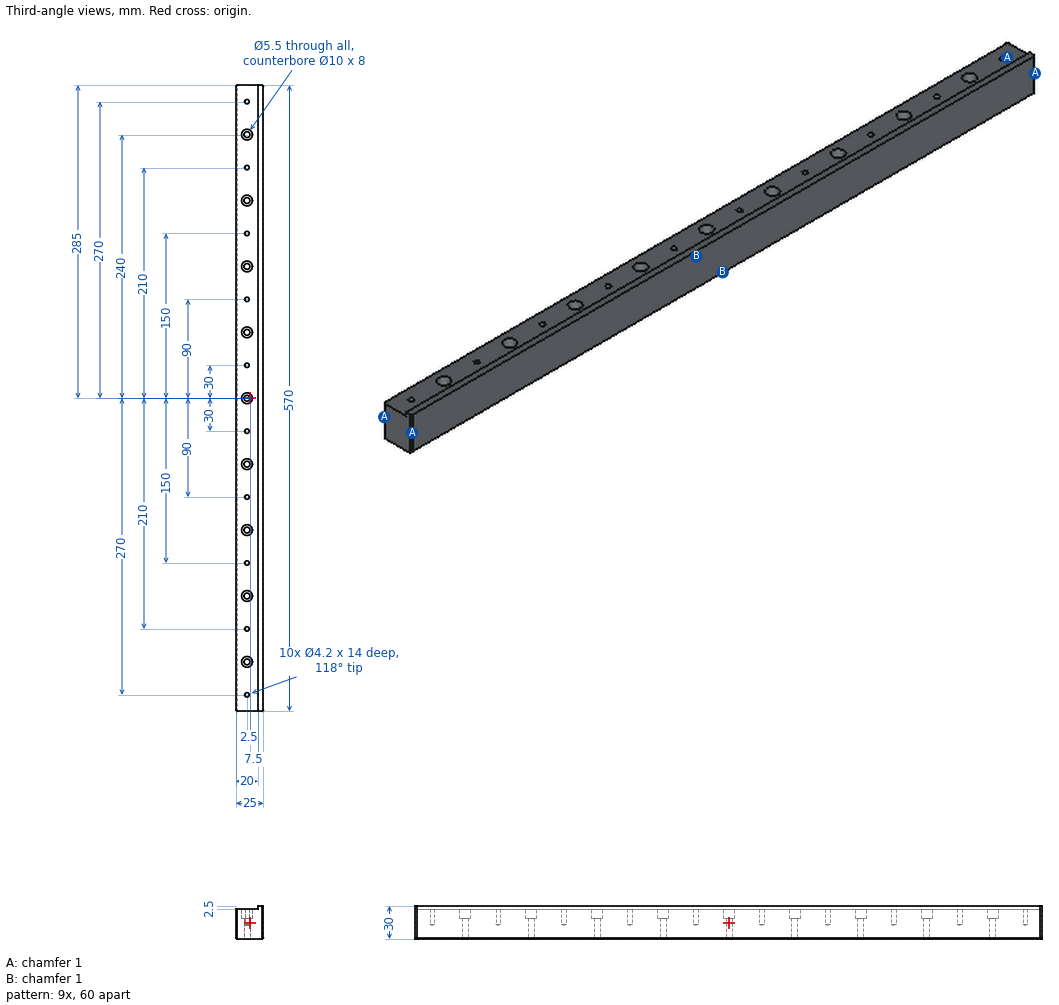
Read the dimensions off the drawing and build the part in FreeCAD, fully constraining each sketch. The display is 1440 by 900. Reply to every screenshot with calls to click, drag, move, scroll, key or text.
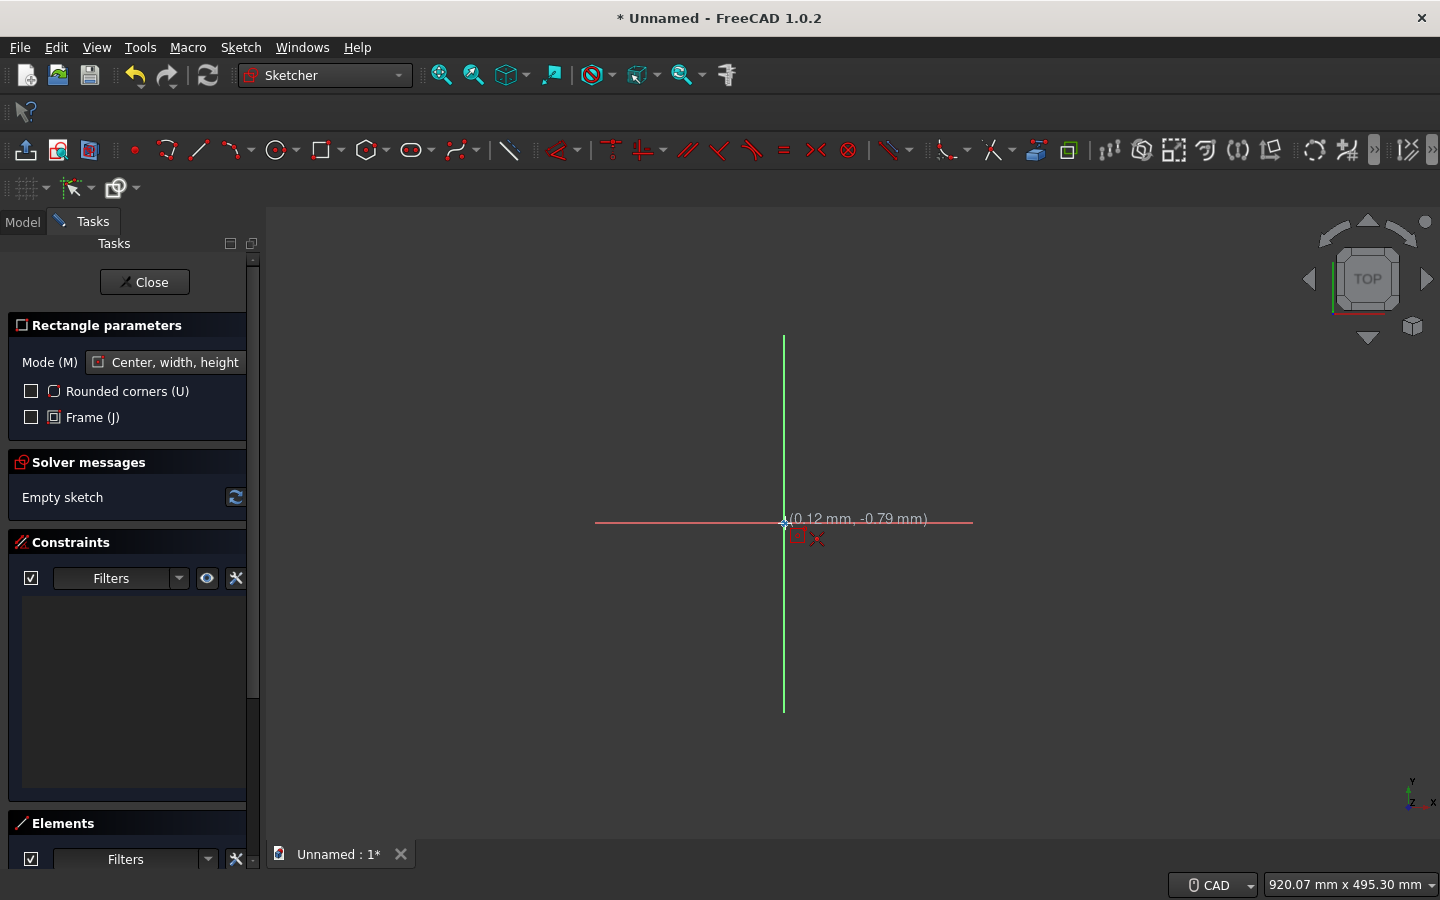
click(784, 523)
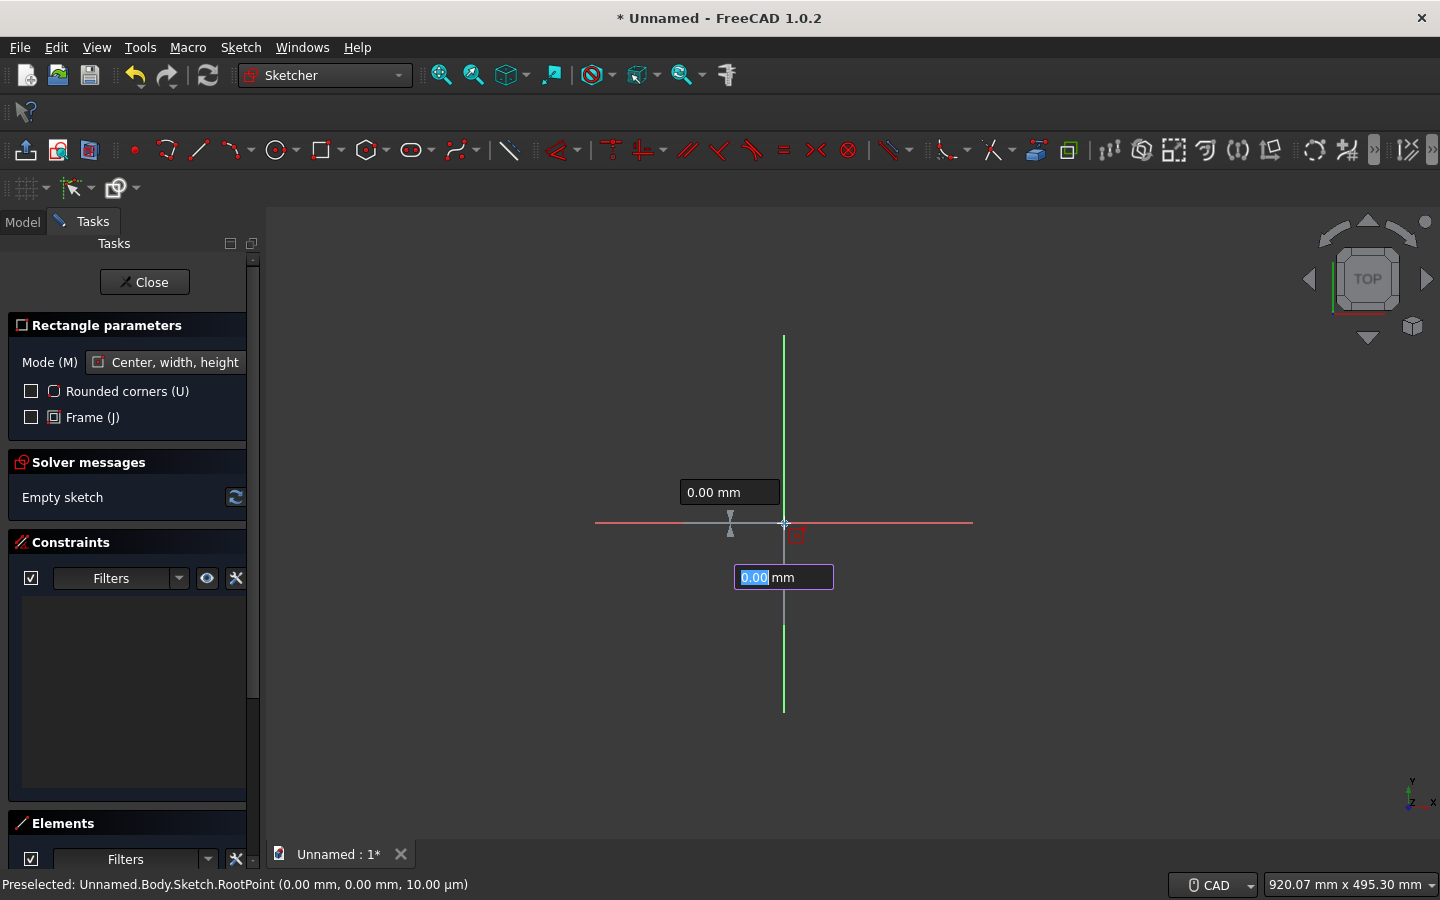
scroll(785, 523, down, 3)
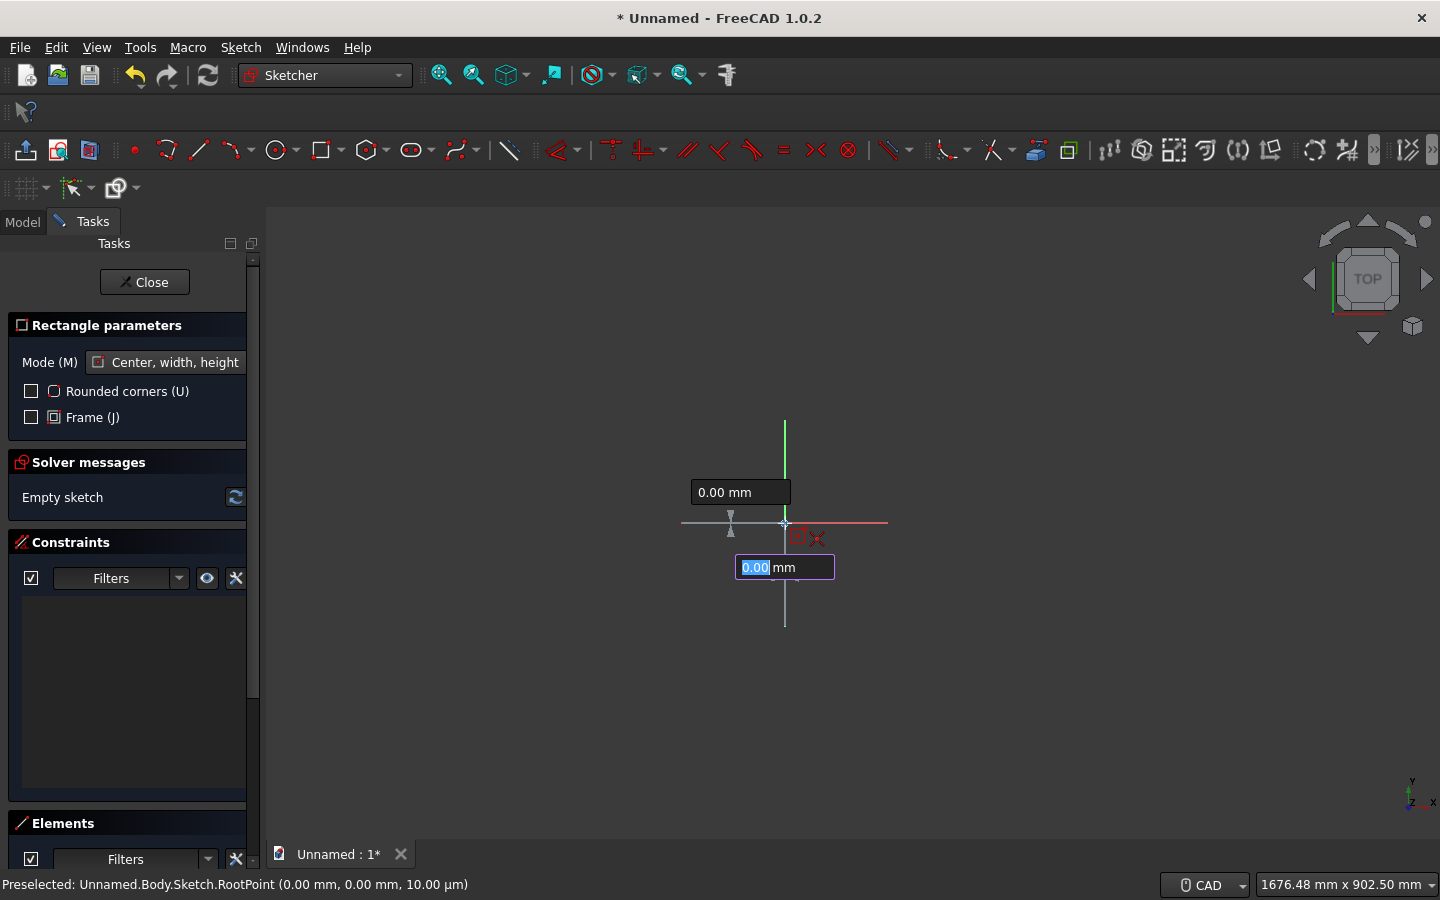
scroll(794, 324, up, 3)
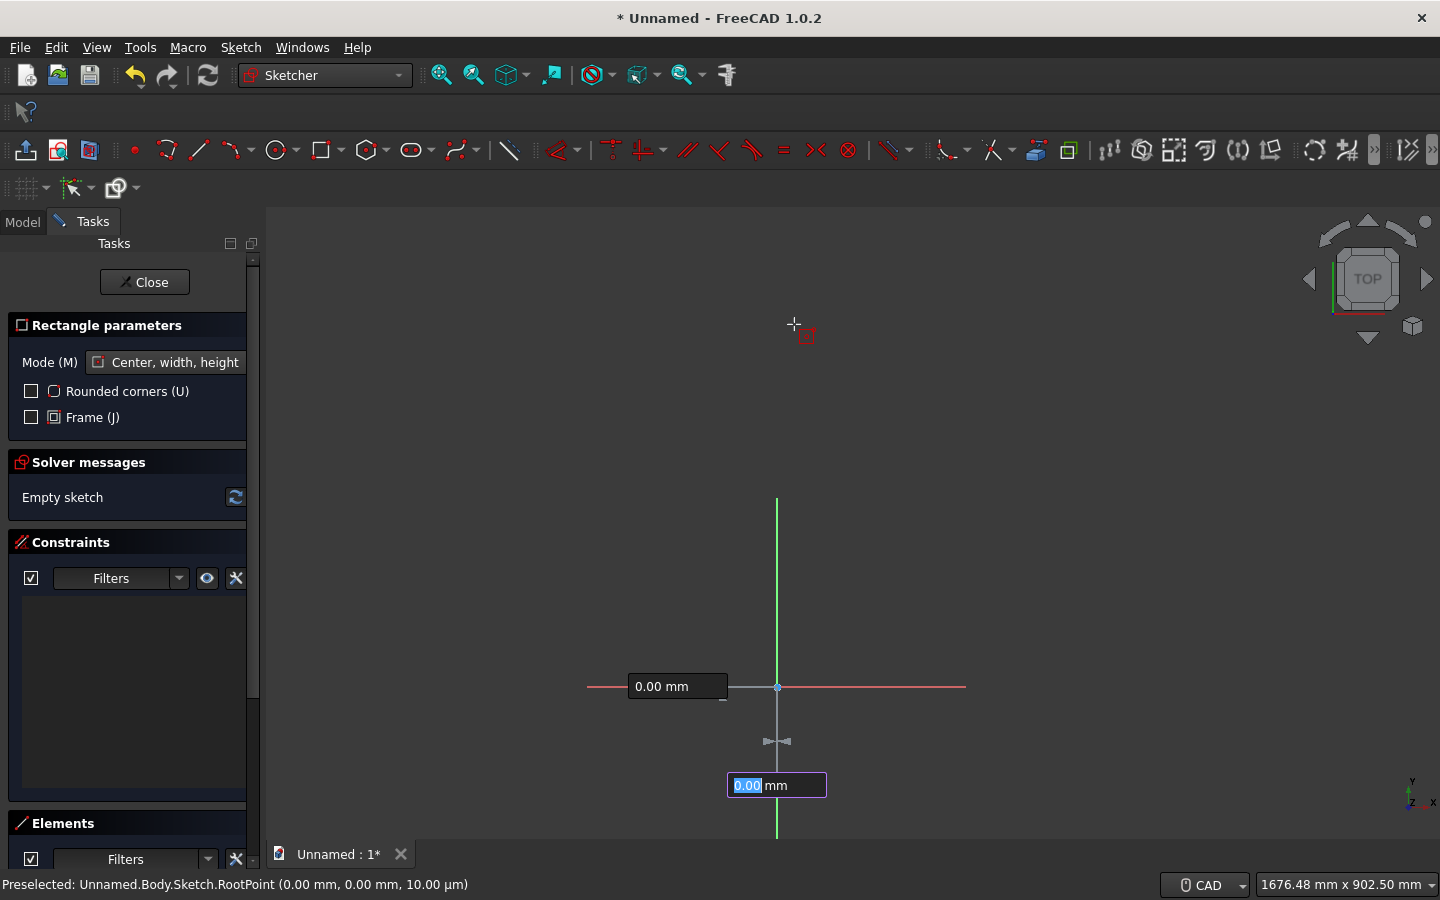
click(793, 324)
key(Escape)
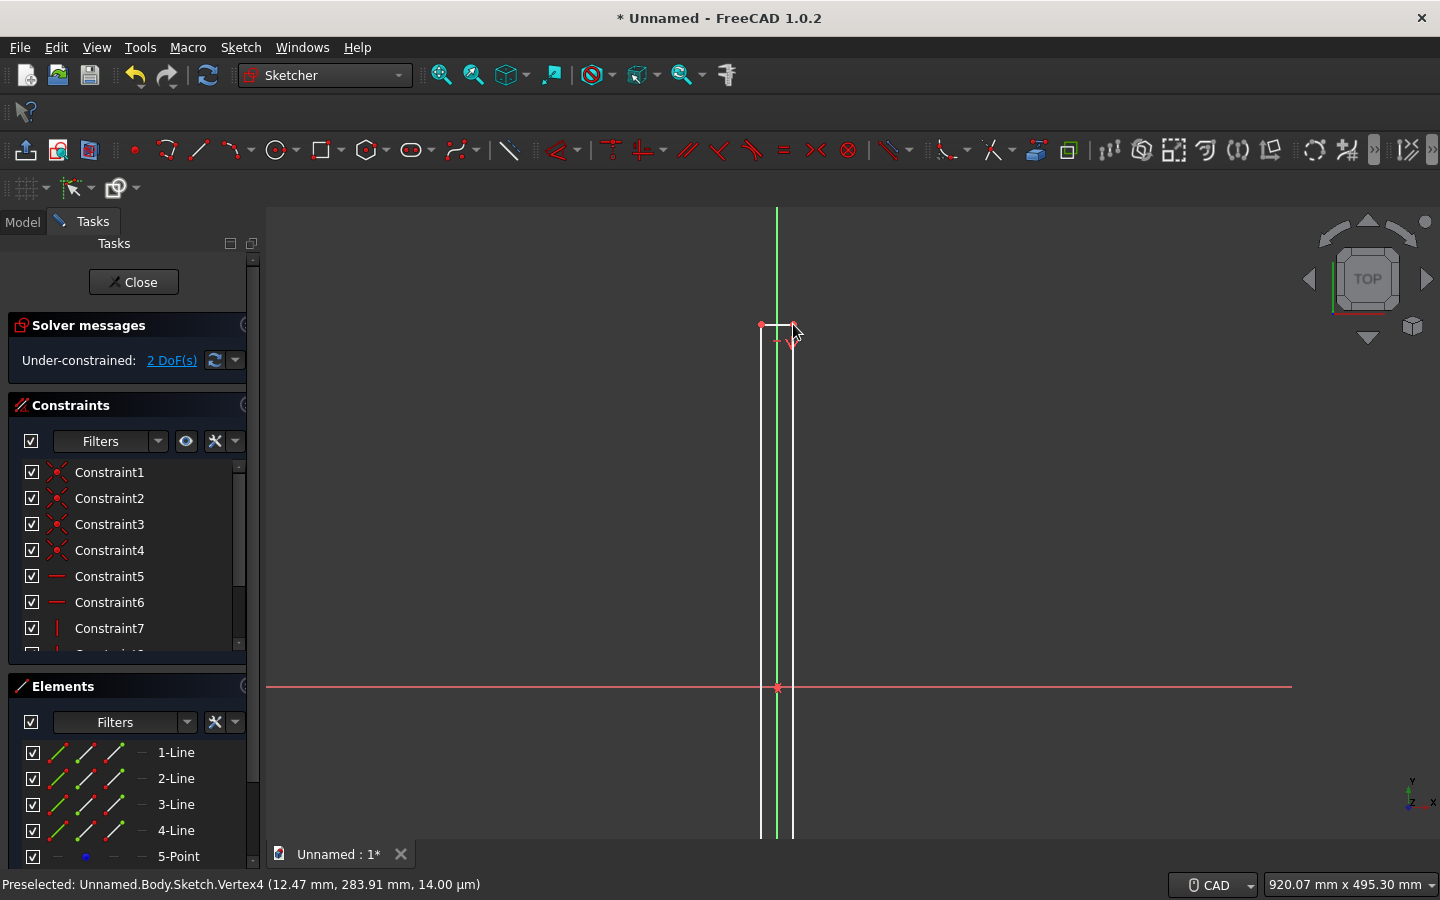
key(d)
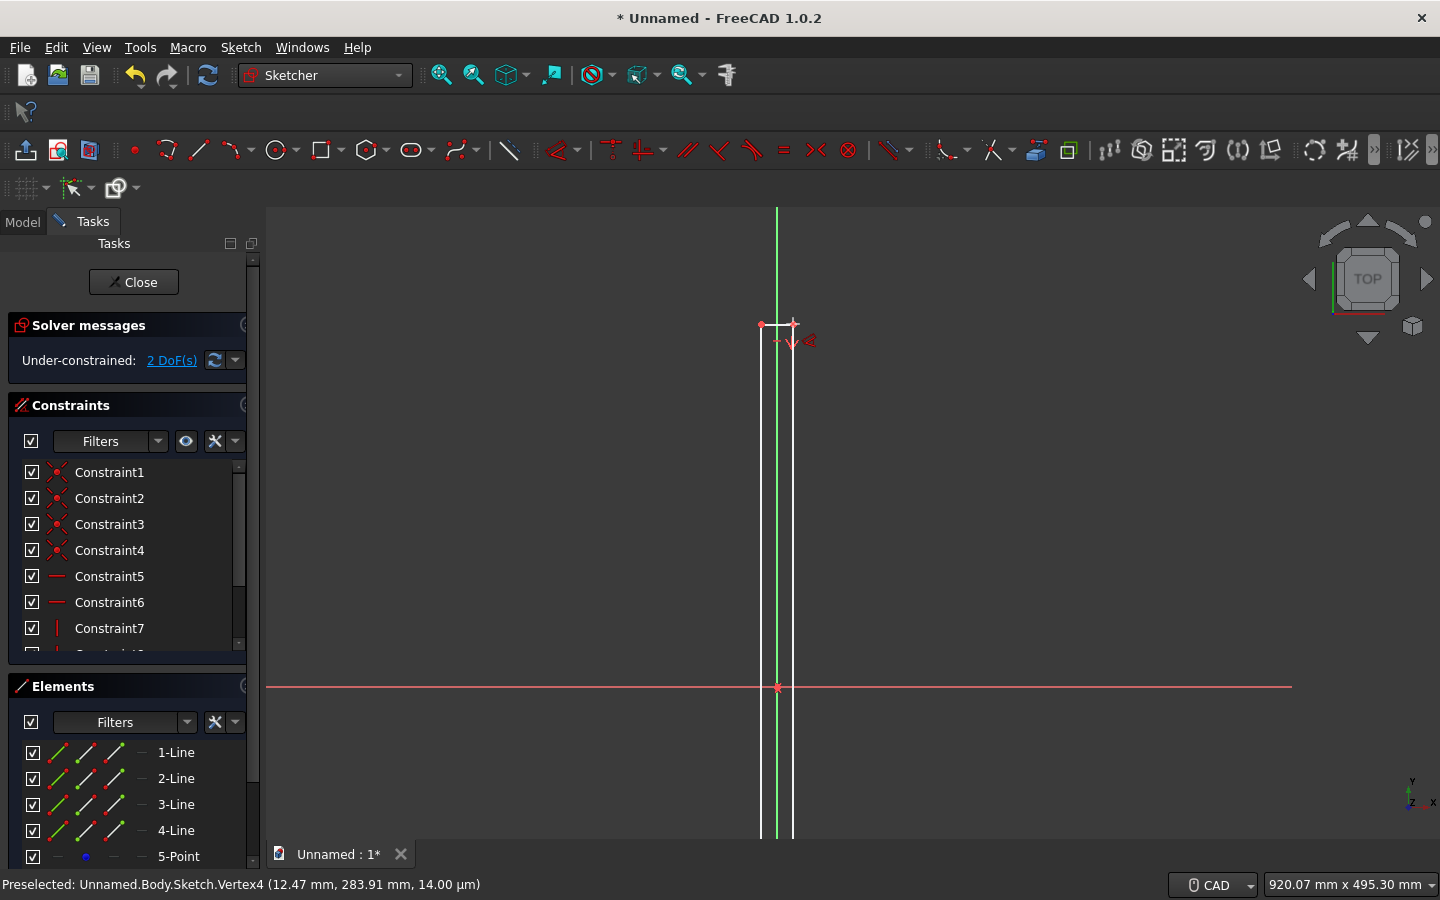
scroll(794, 323, down, 3)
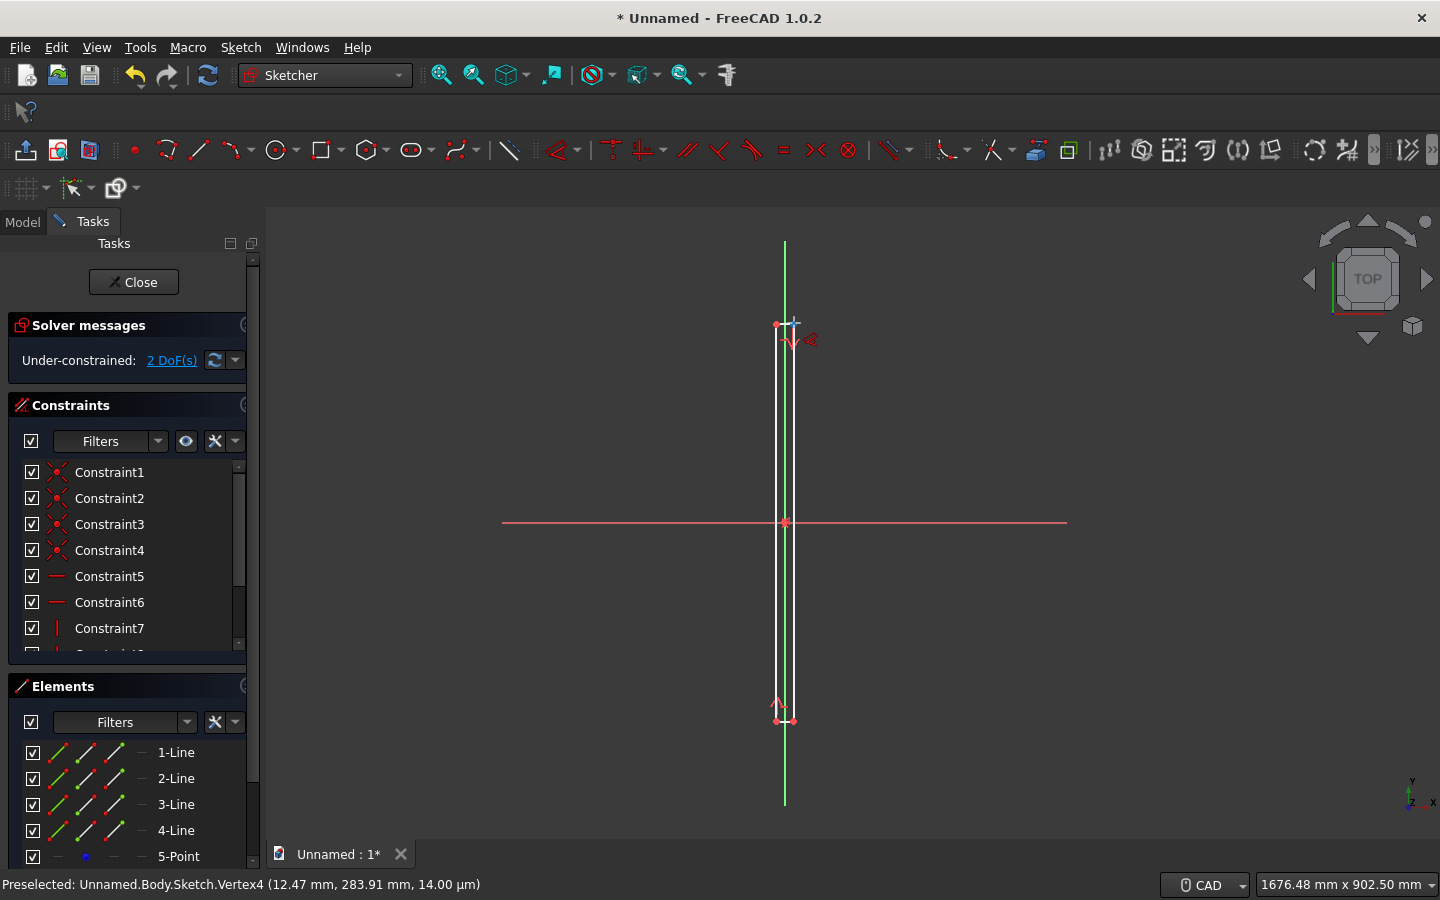
scroll(783, 722, up, 5)